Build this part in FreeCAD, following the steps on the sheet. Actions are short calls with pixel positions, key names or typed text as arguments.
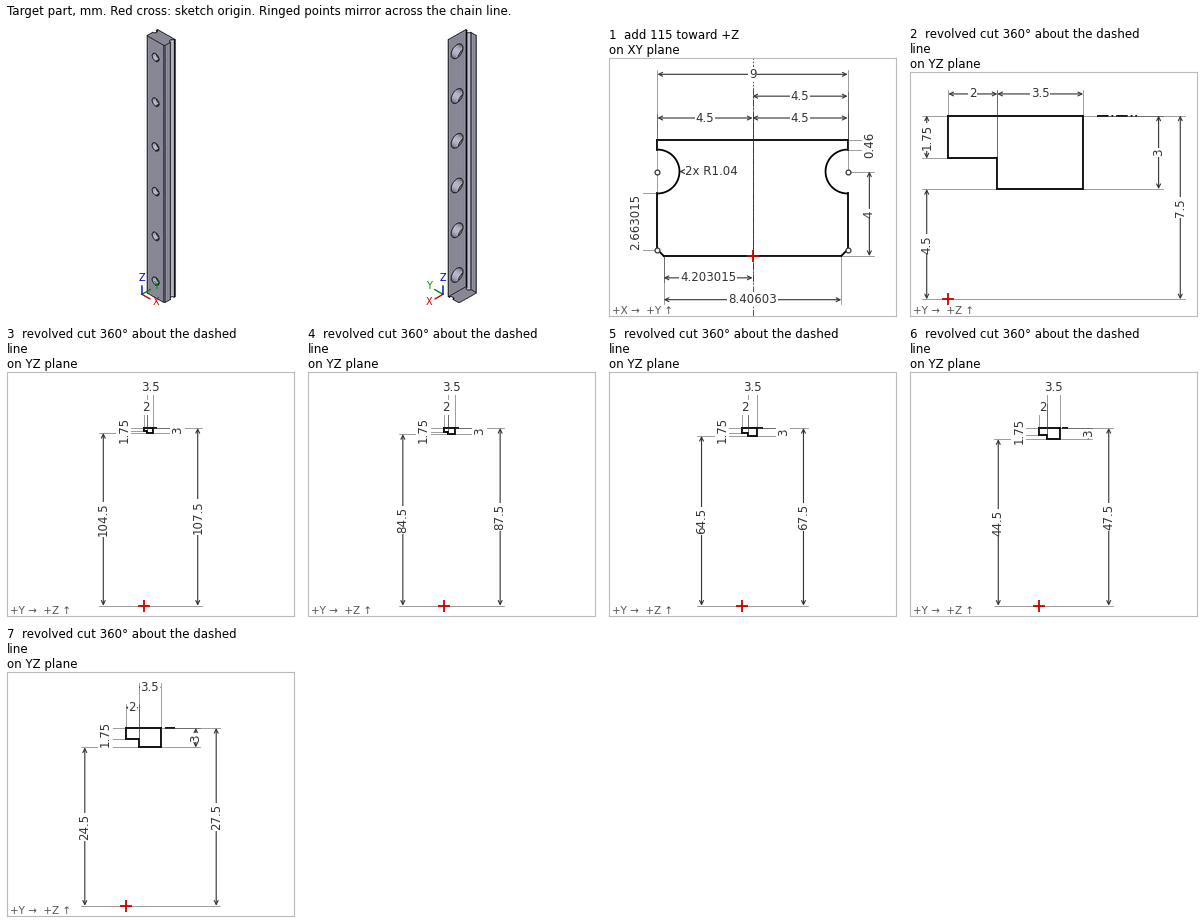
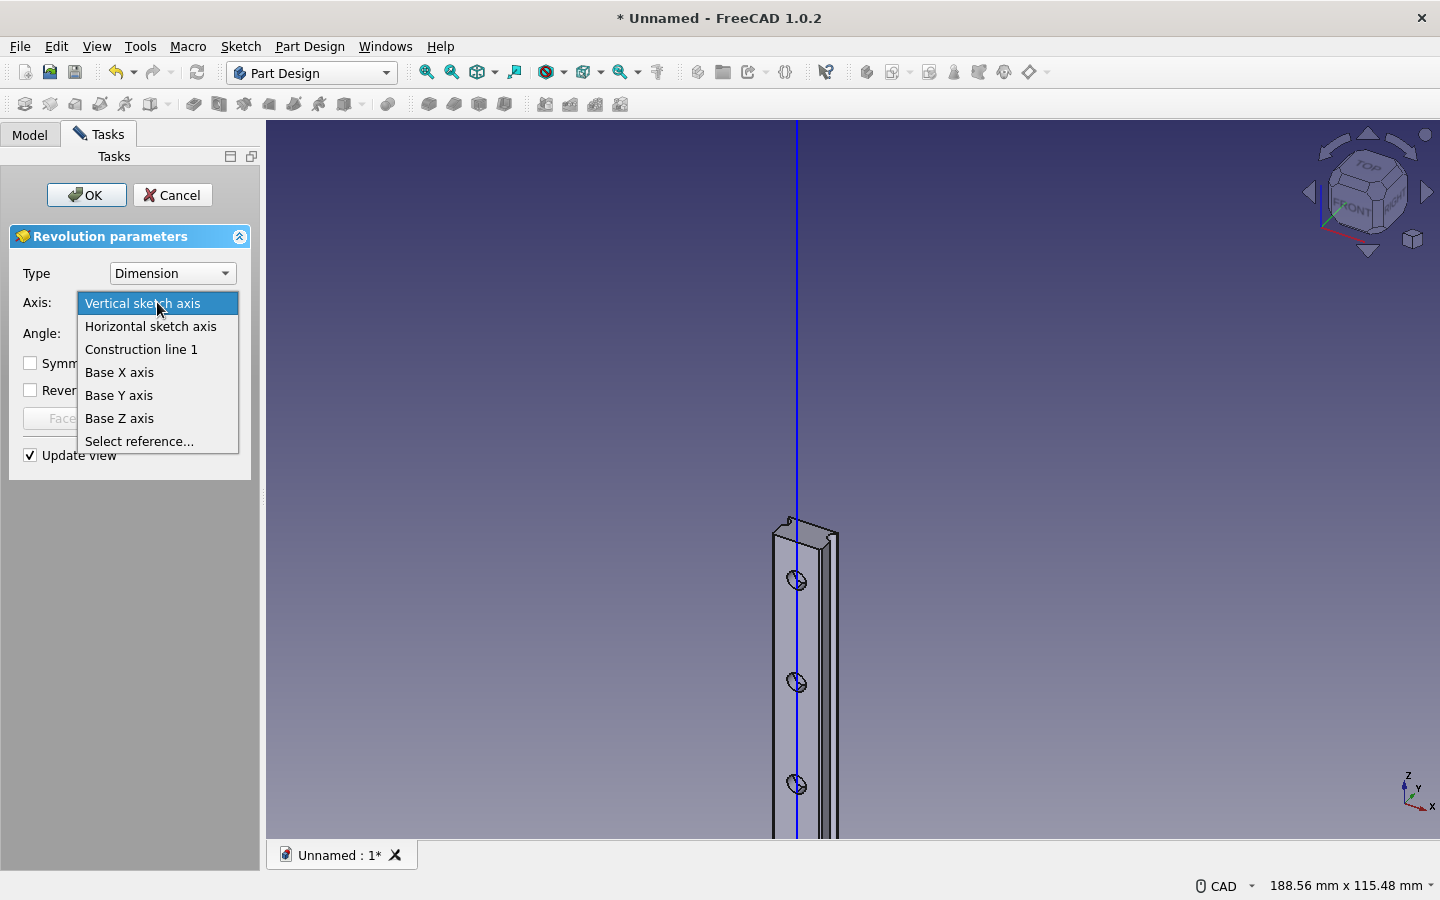
click(156, 350)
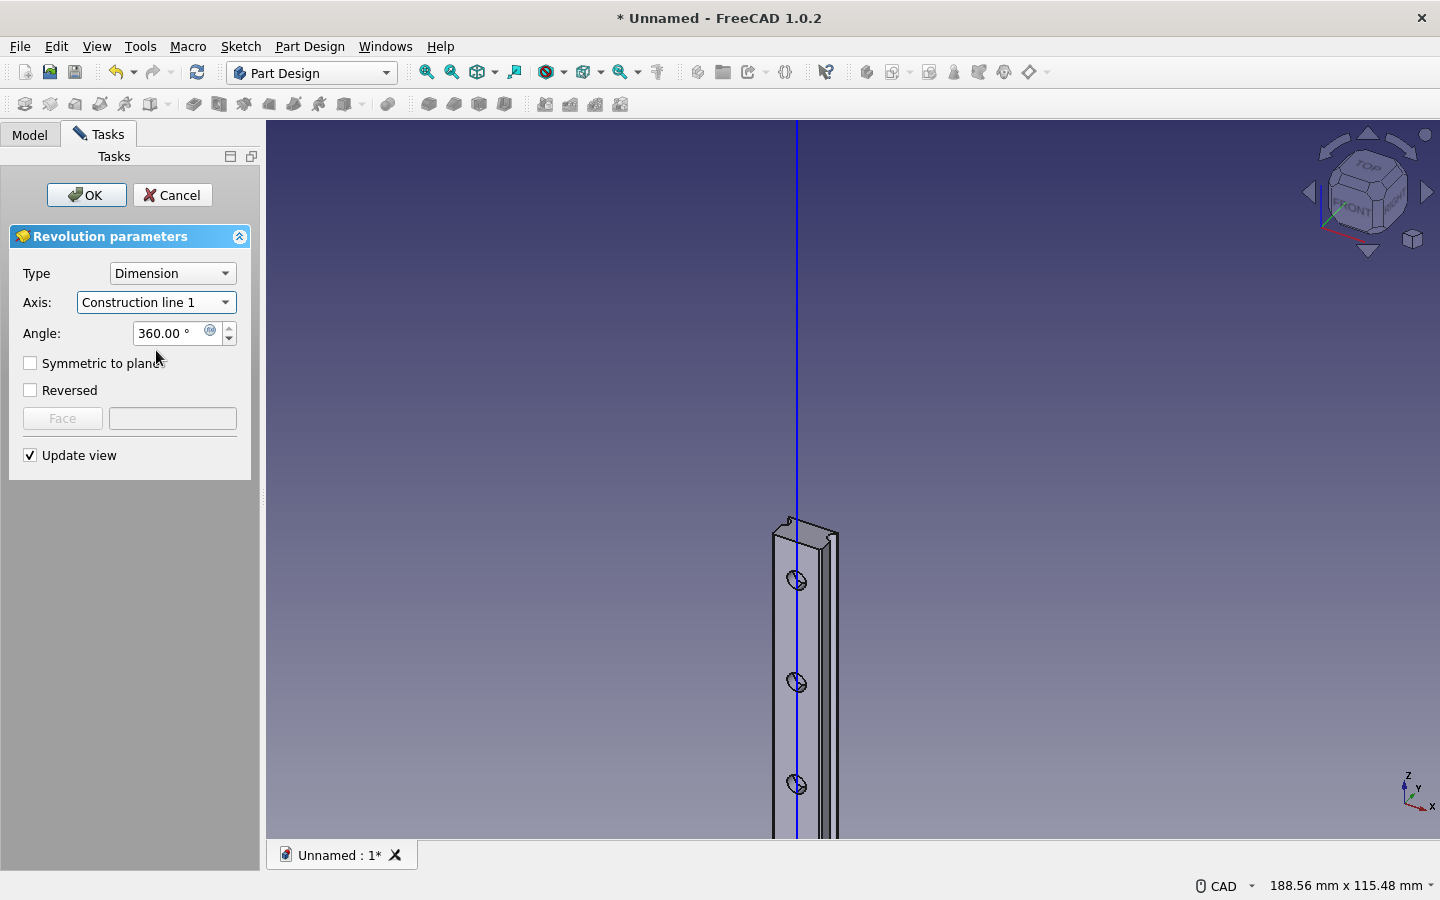
click(87, 195)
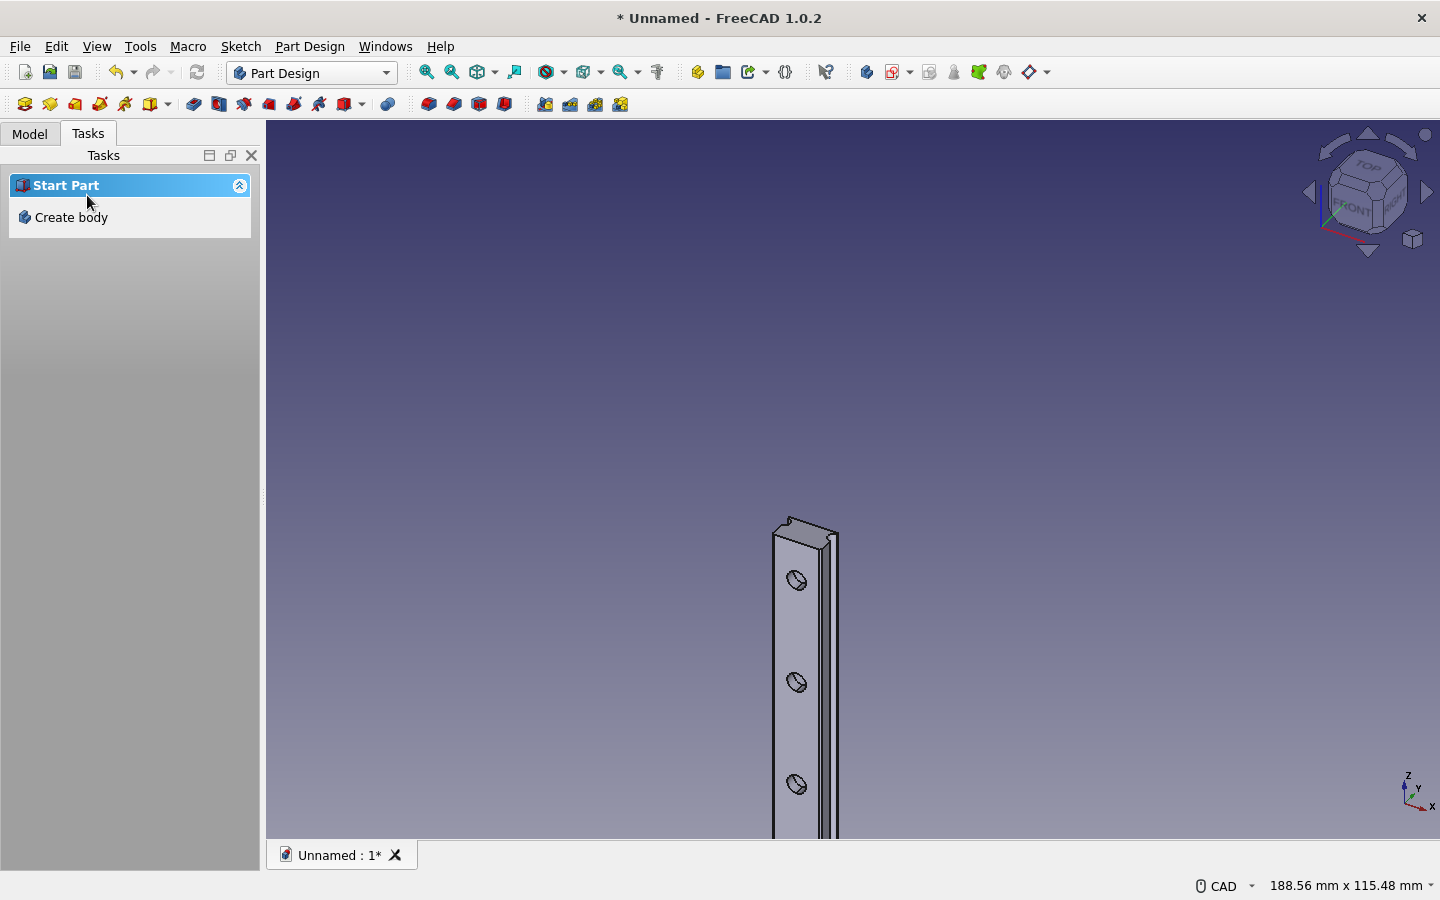
key(v)
key(f)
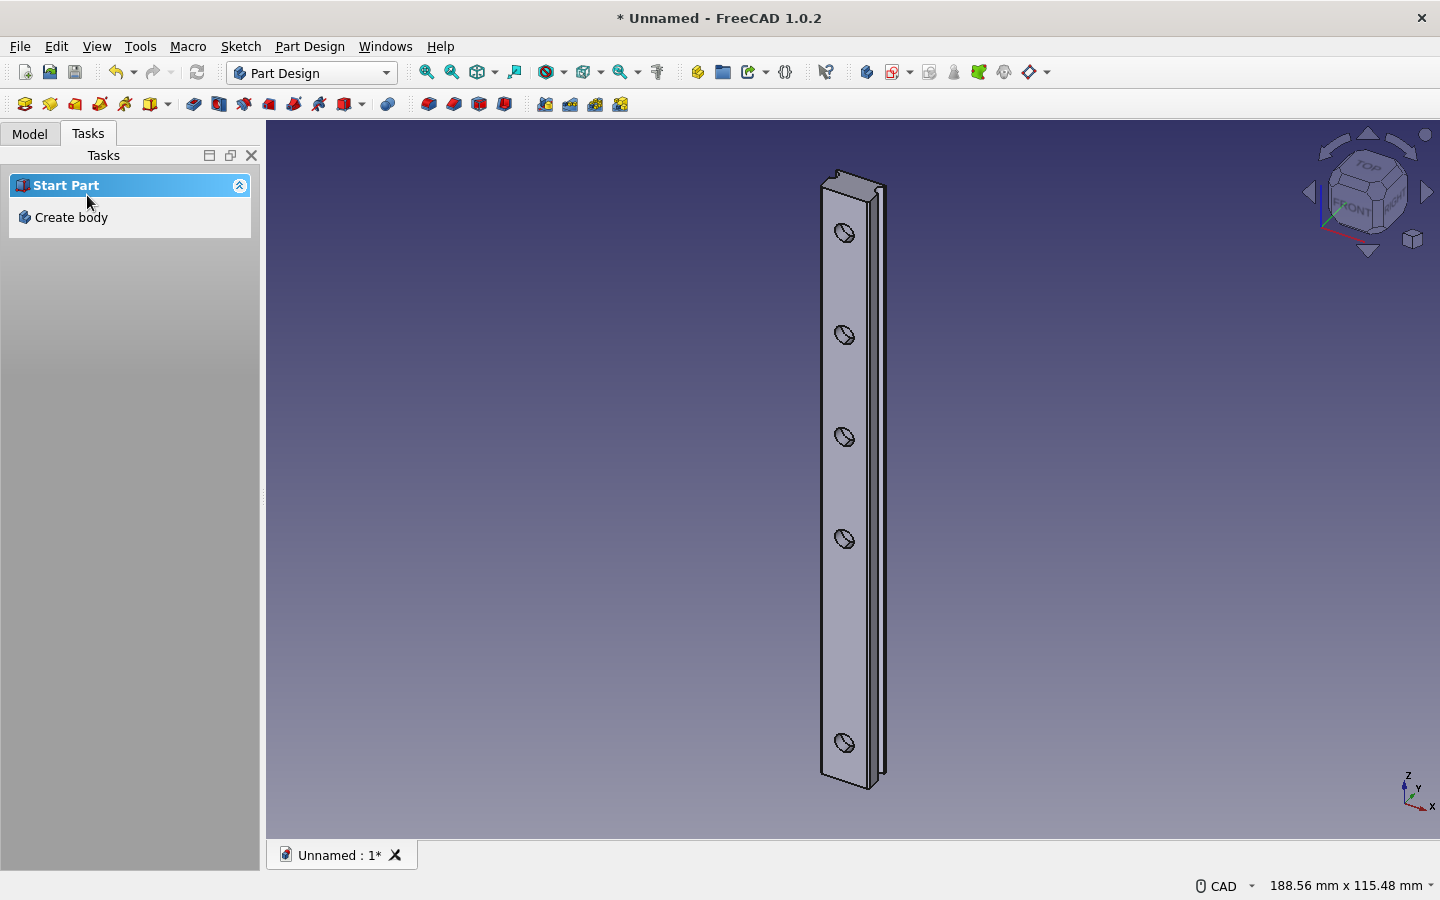
click(892, 72)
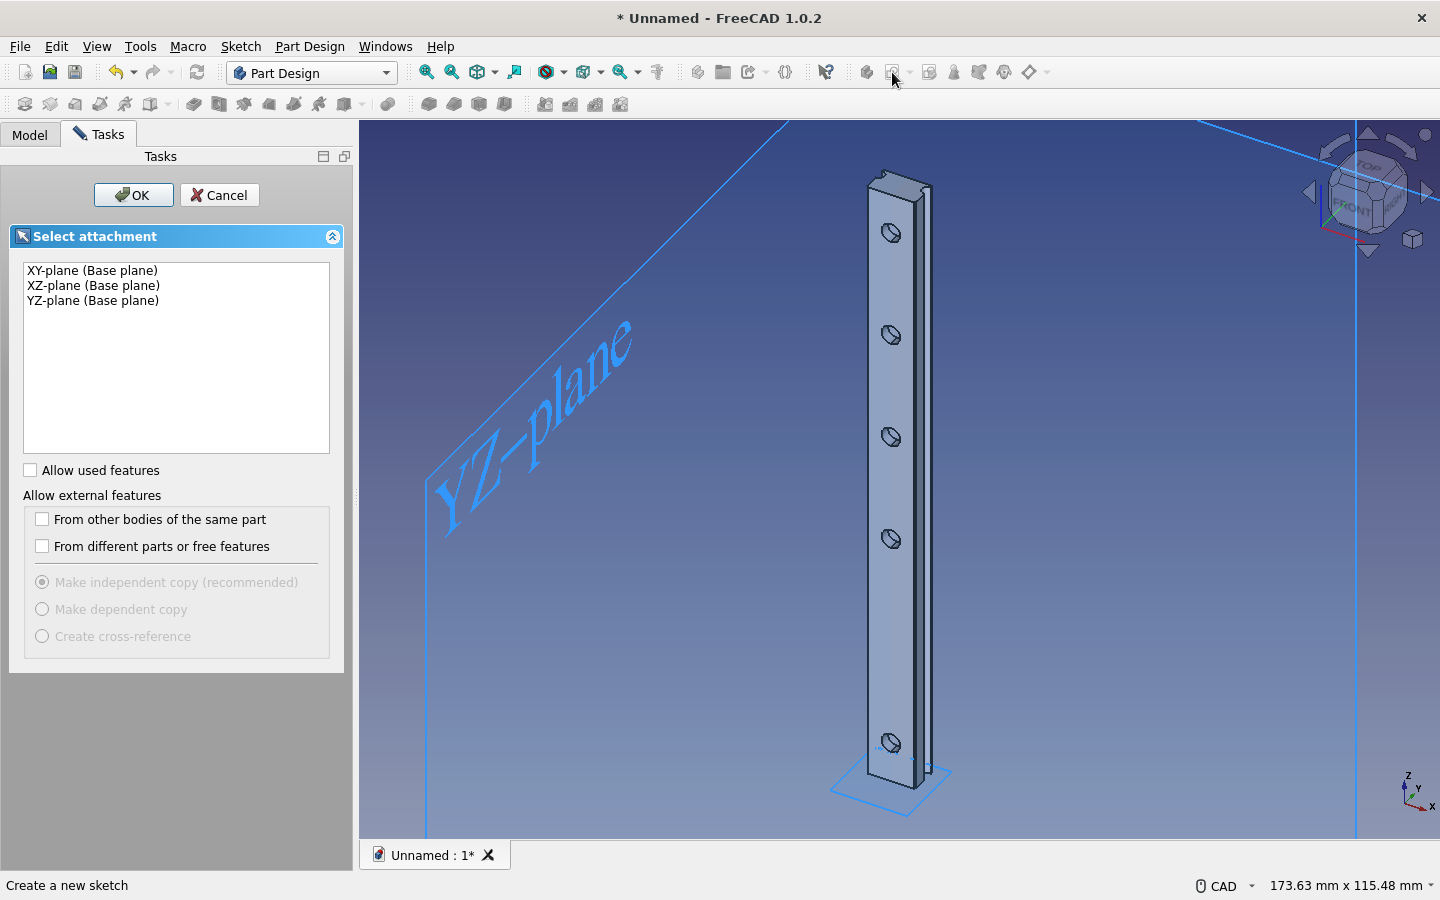
click(84, 300)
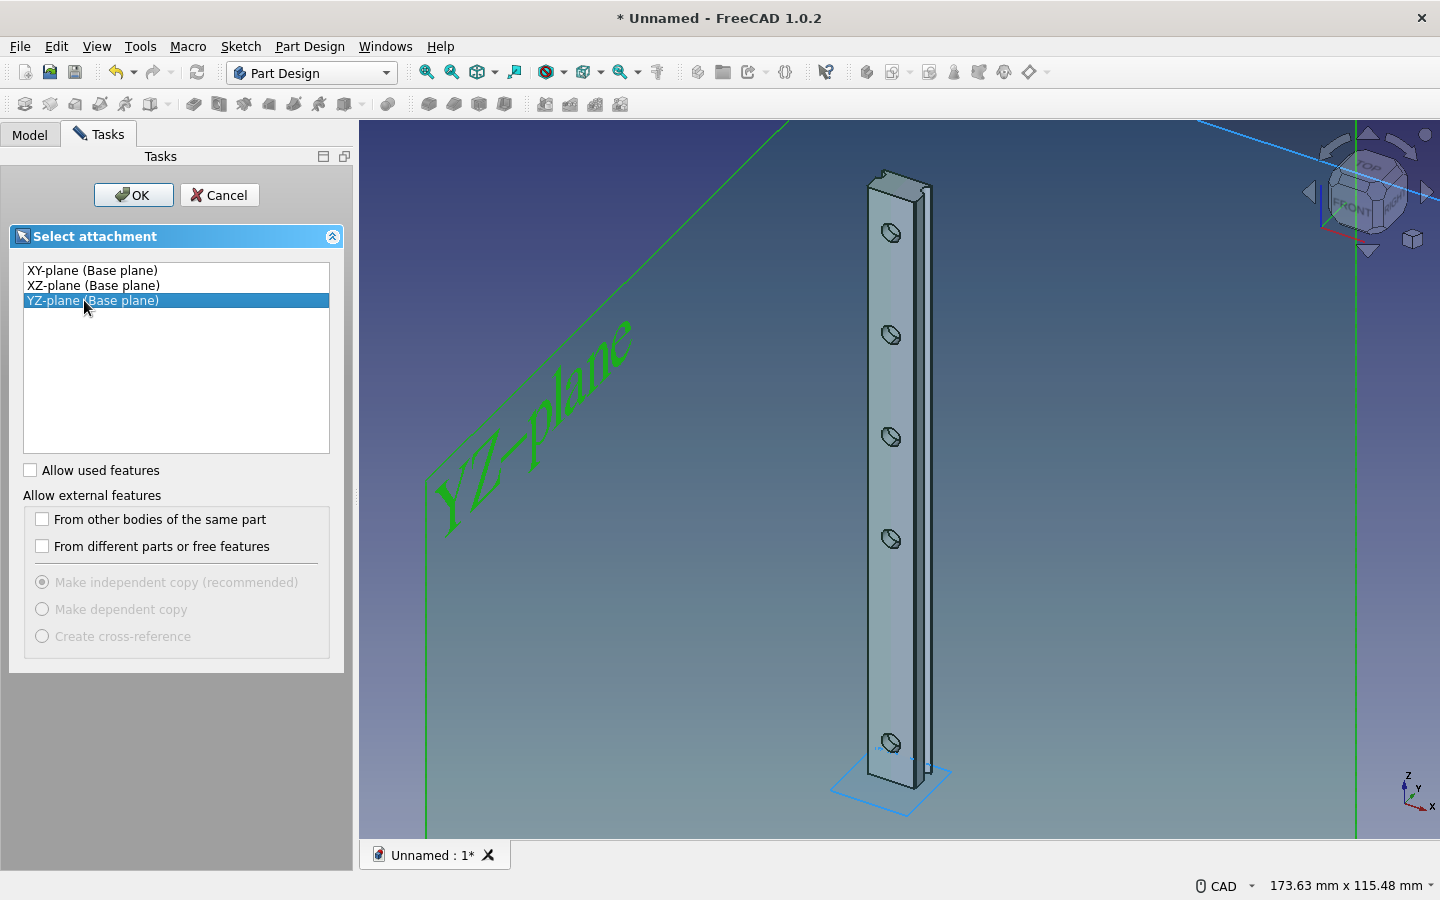
click(134, 195)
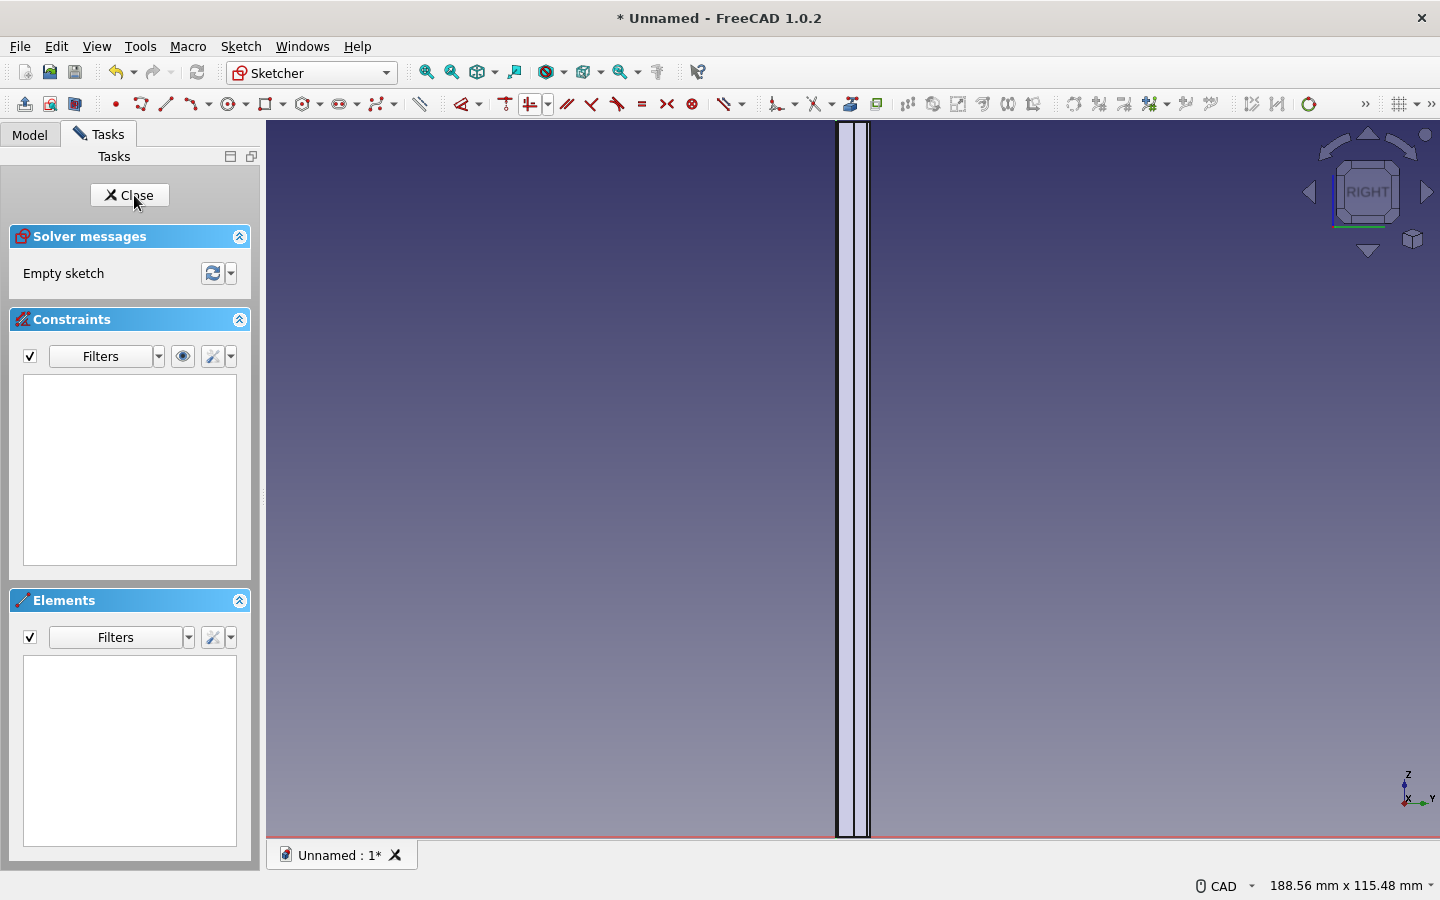
key(q)
key(s)